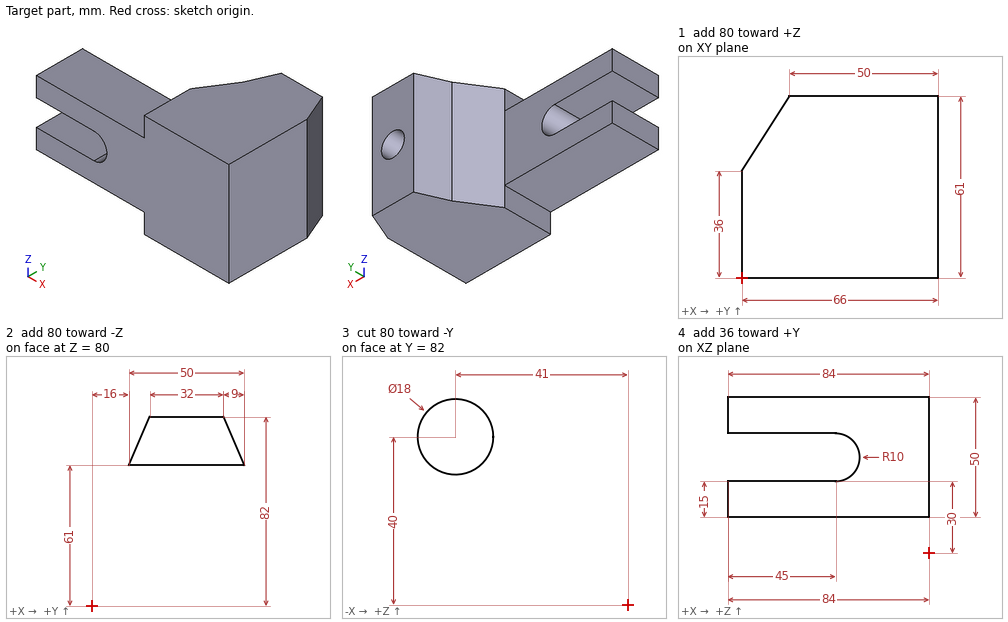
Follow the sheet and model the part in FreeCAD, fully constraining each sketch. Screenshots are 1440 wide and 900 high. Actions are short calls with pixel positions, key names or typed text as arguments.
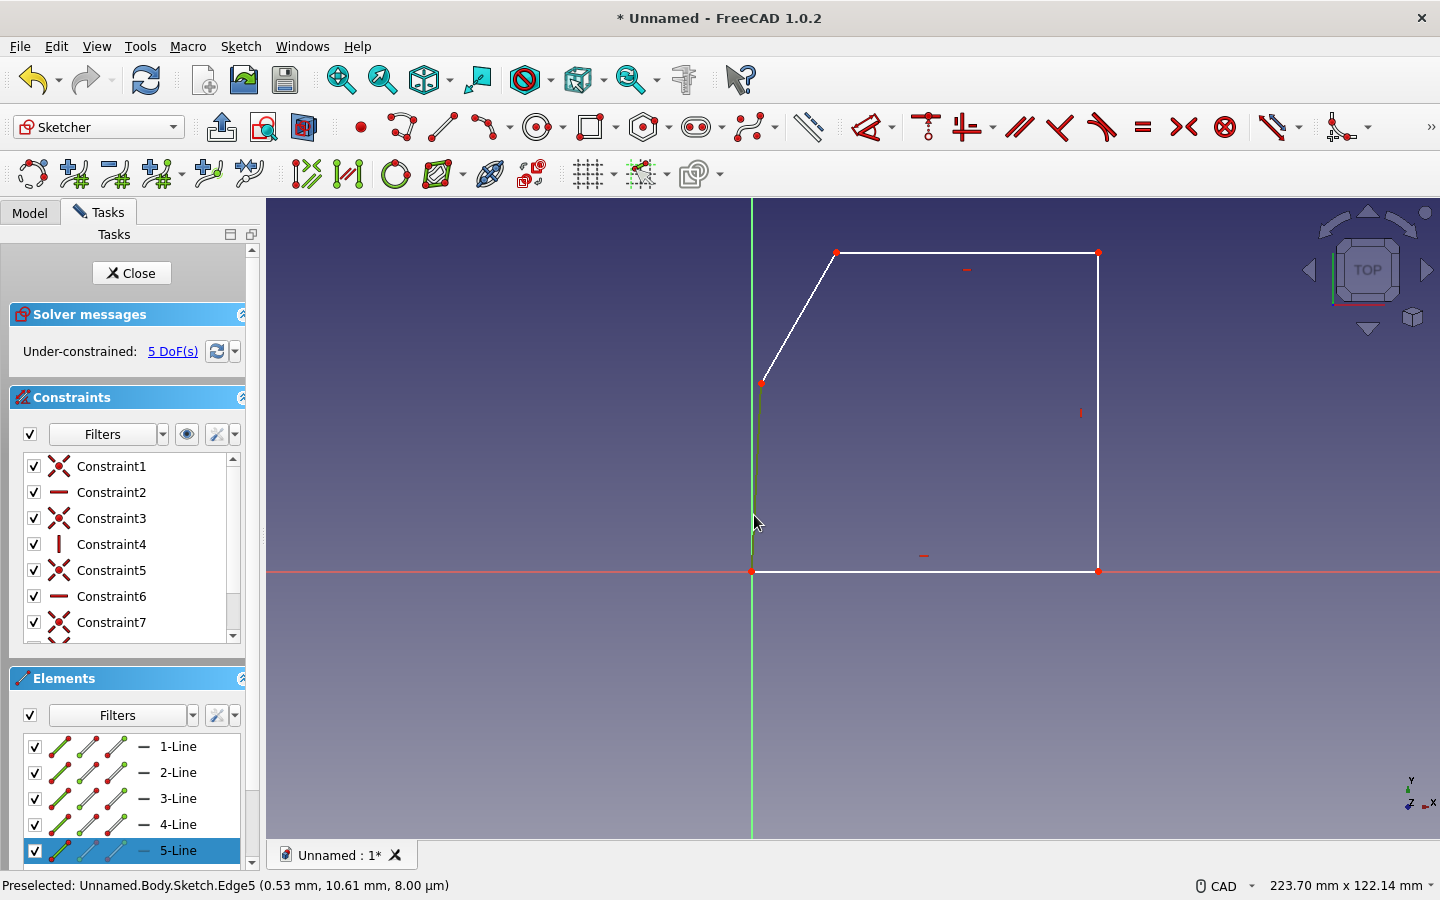
key(v)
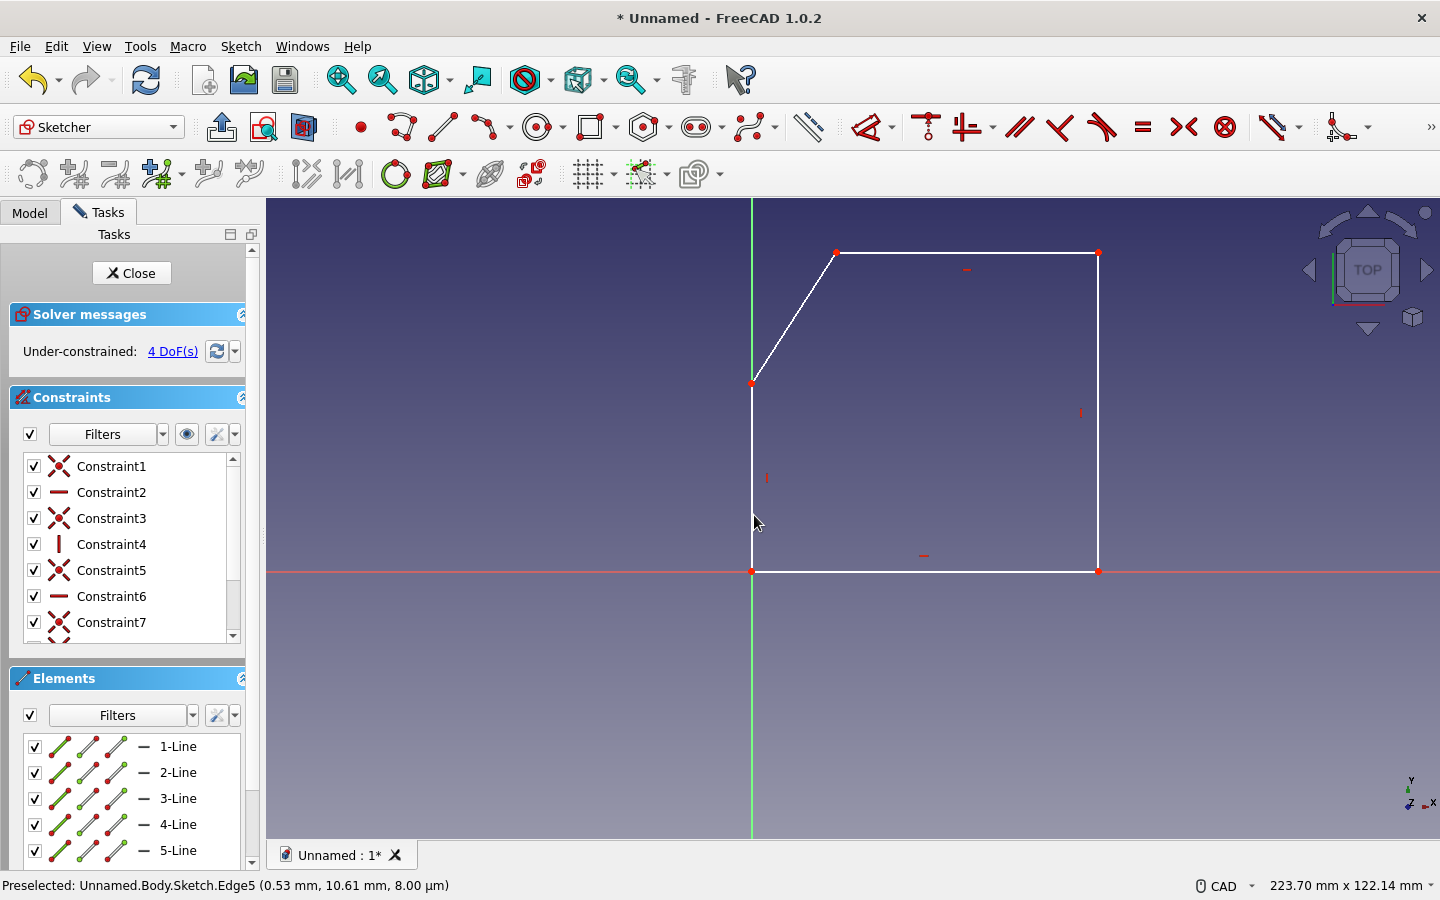
key(d)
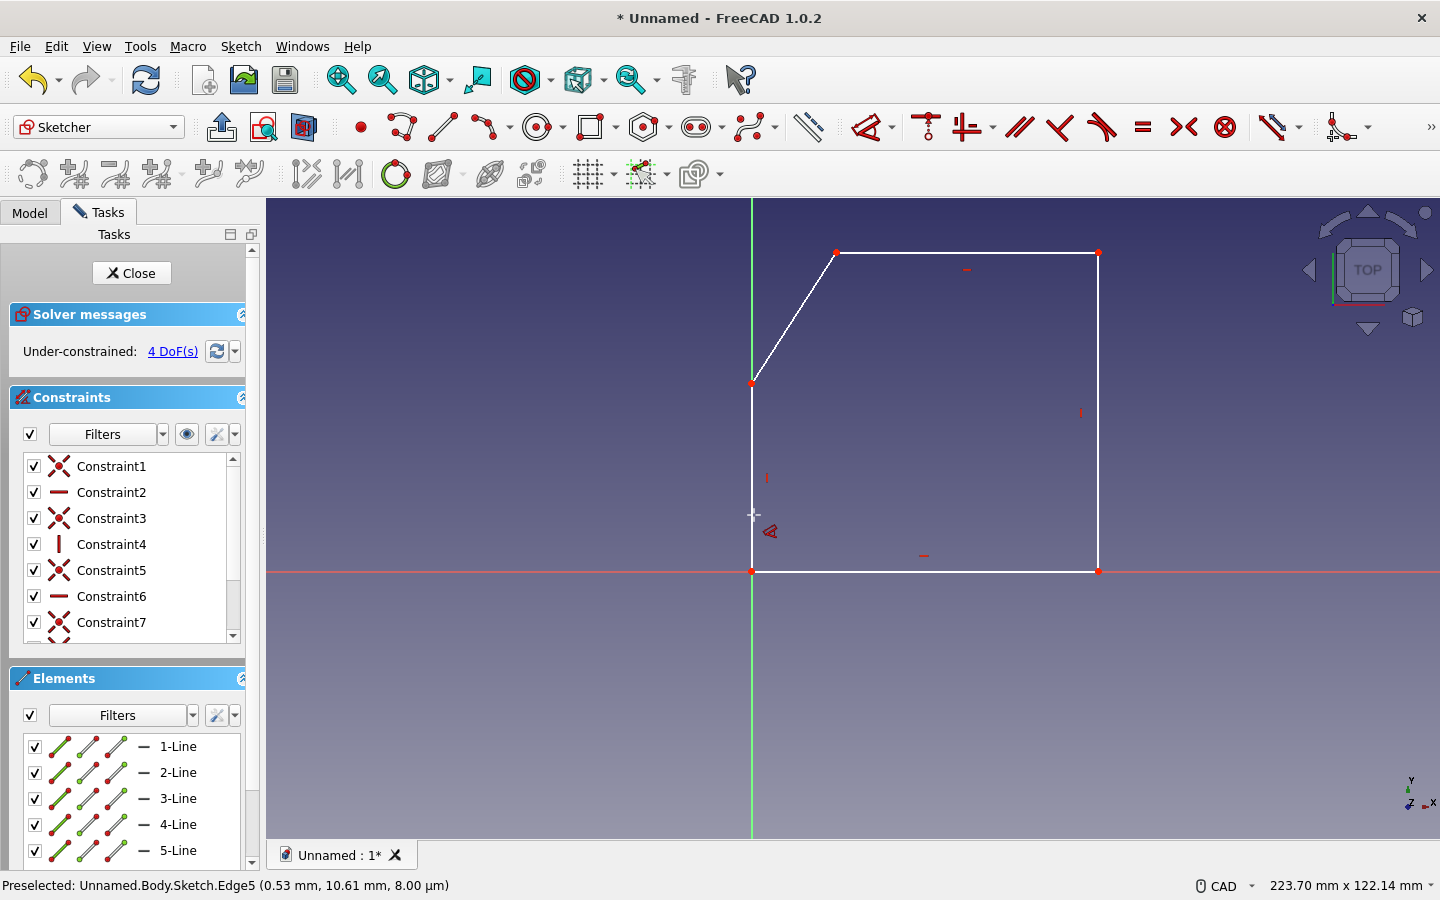
click(856, 572)
click(925, 606)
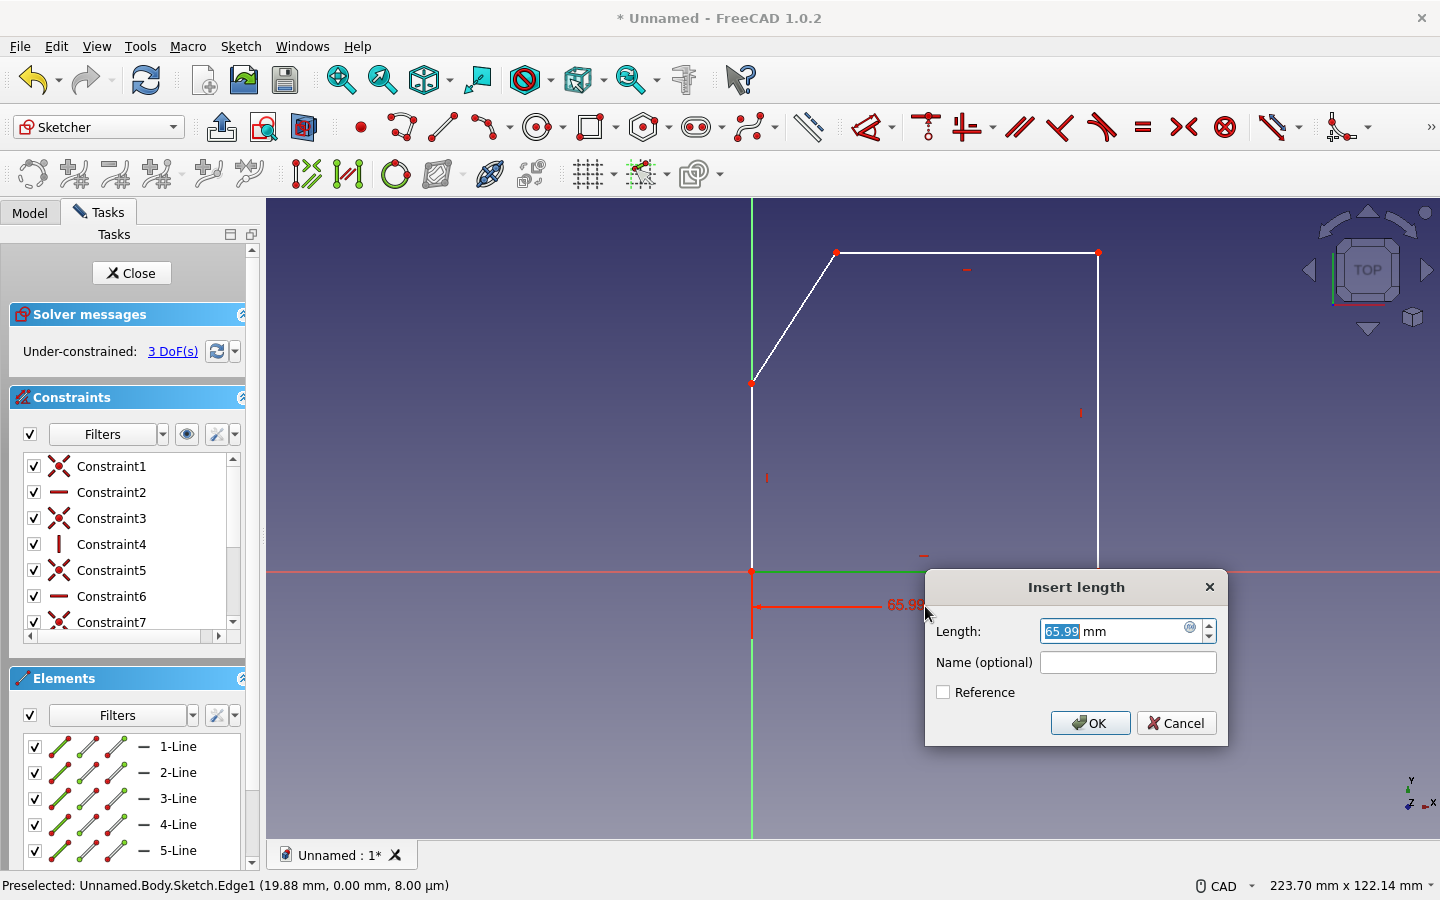
text(66)
key(Return)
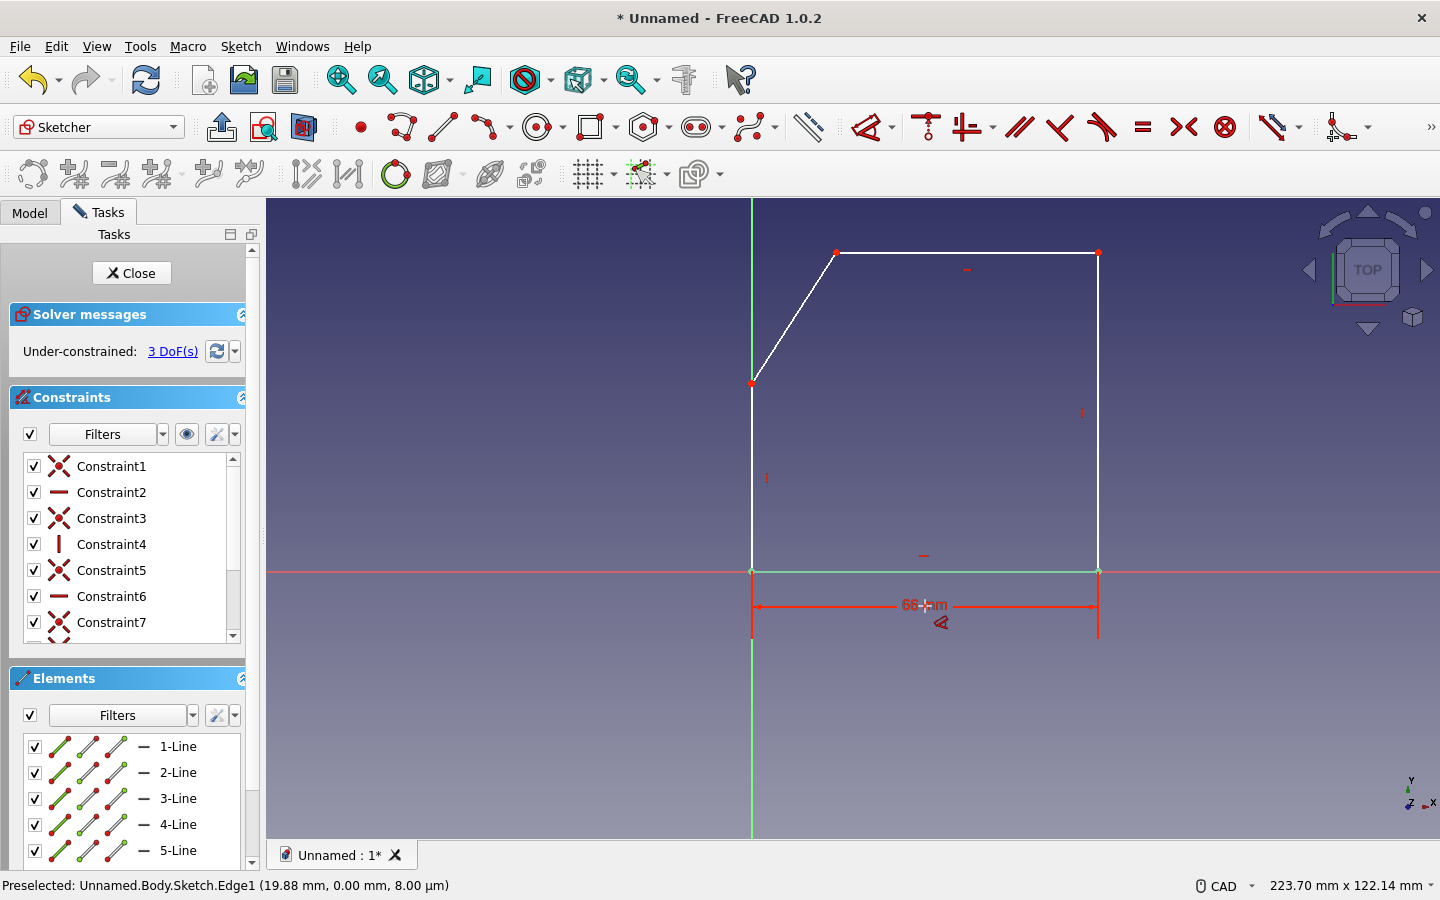
click(1098, 476)
click(1132, 412)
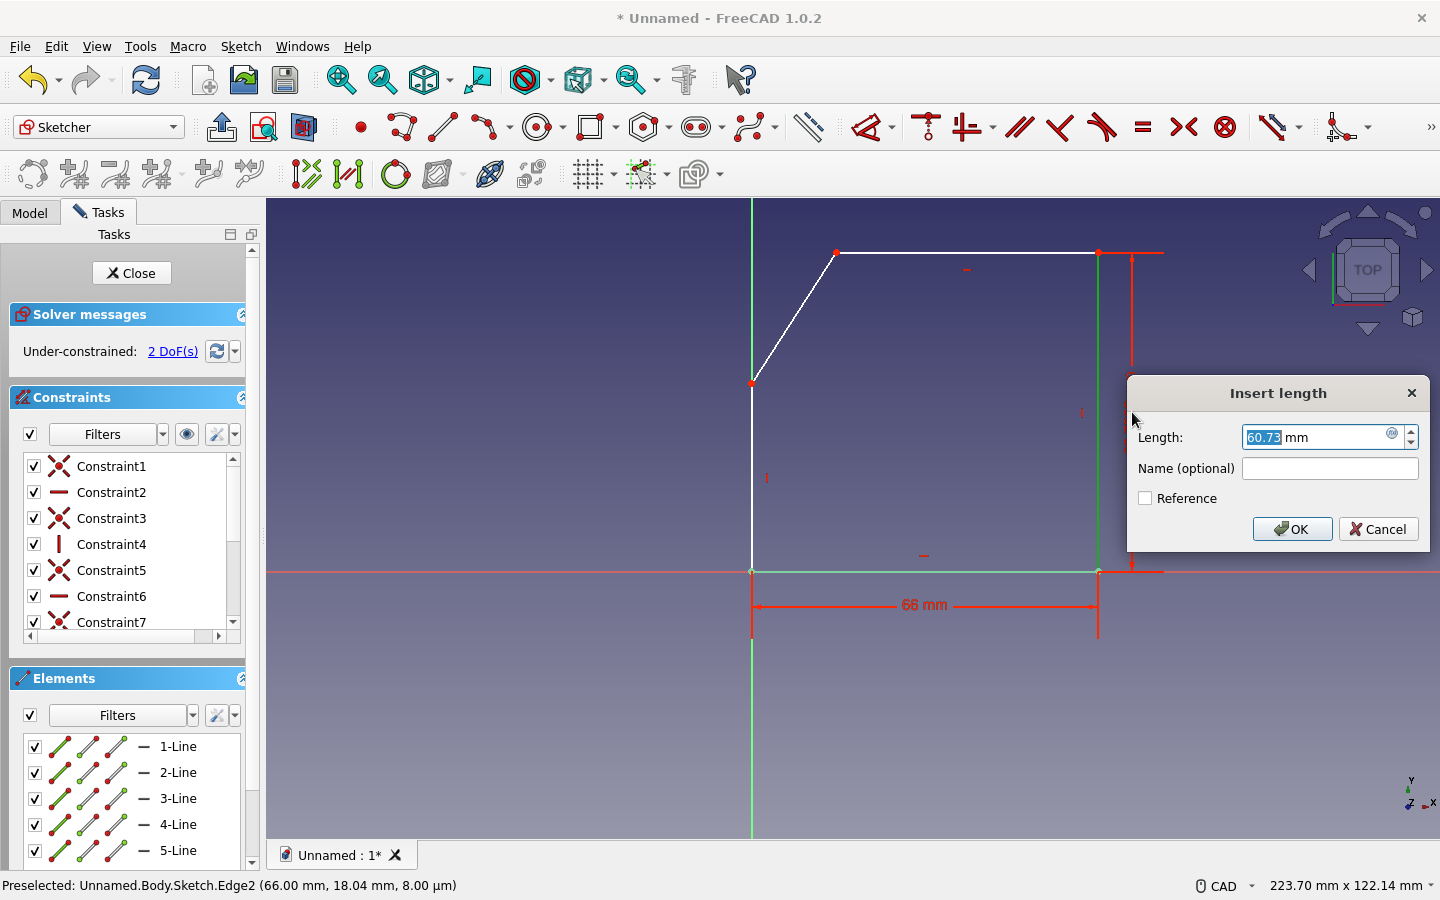
text(61)
key(Return)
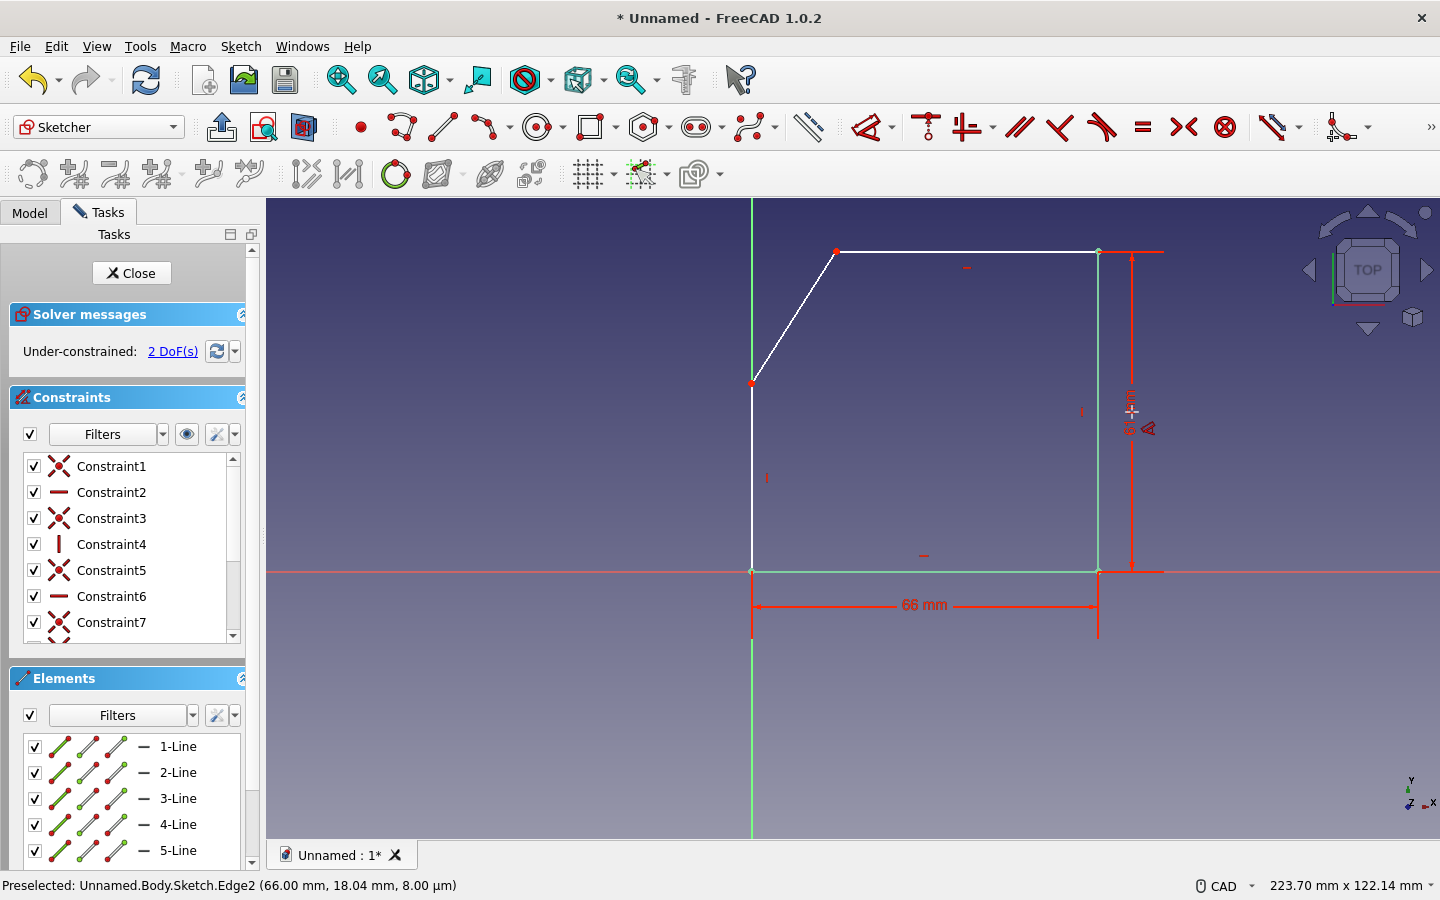
click(1019, 252)
click(967, 286)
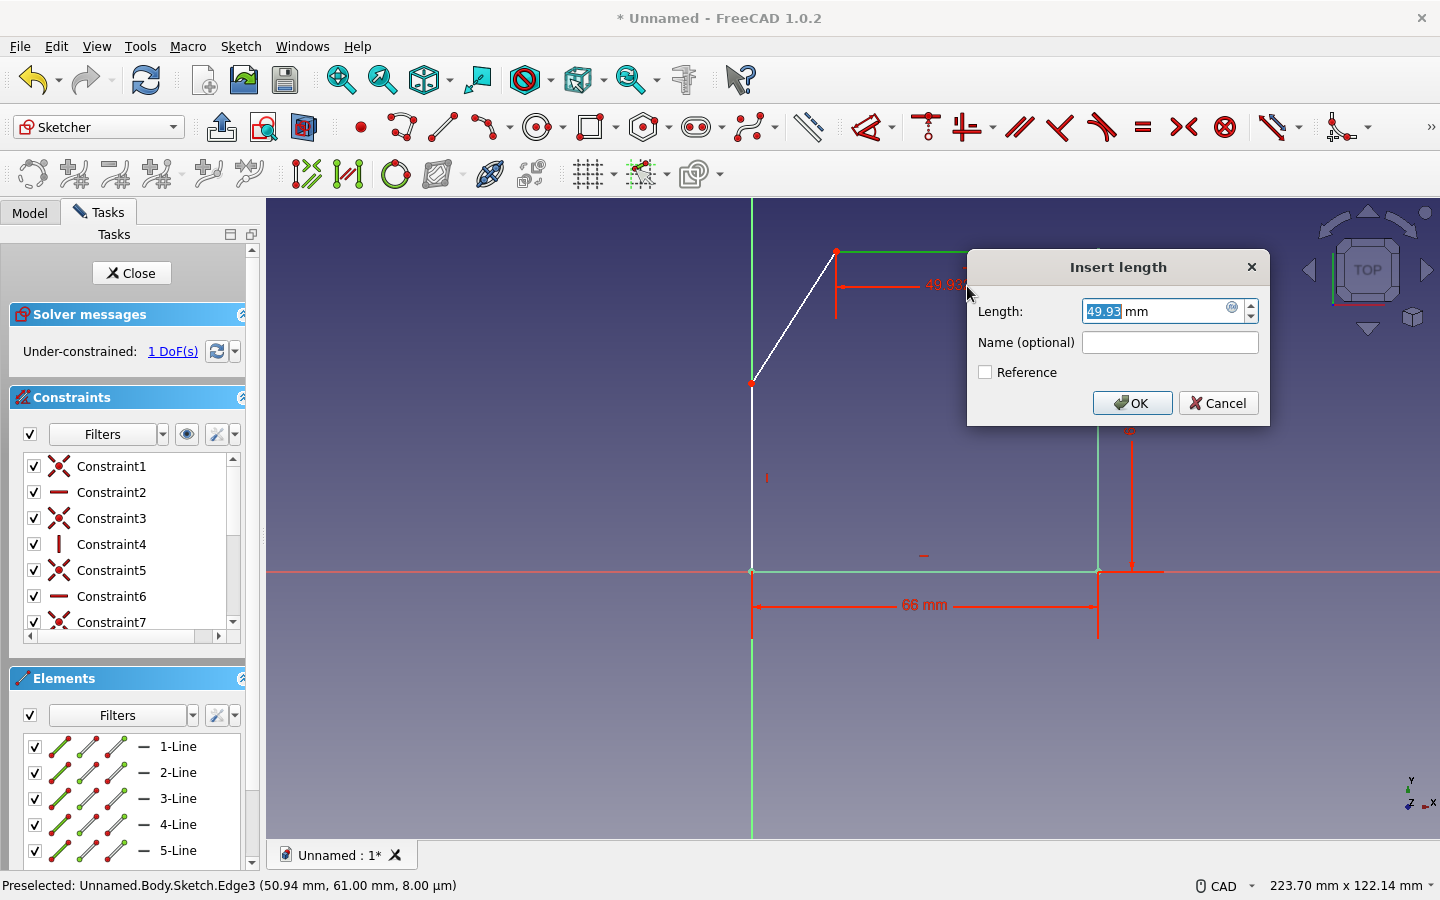
text(50)
key(Return)